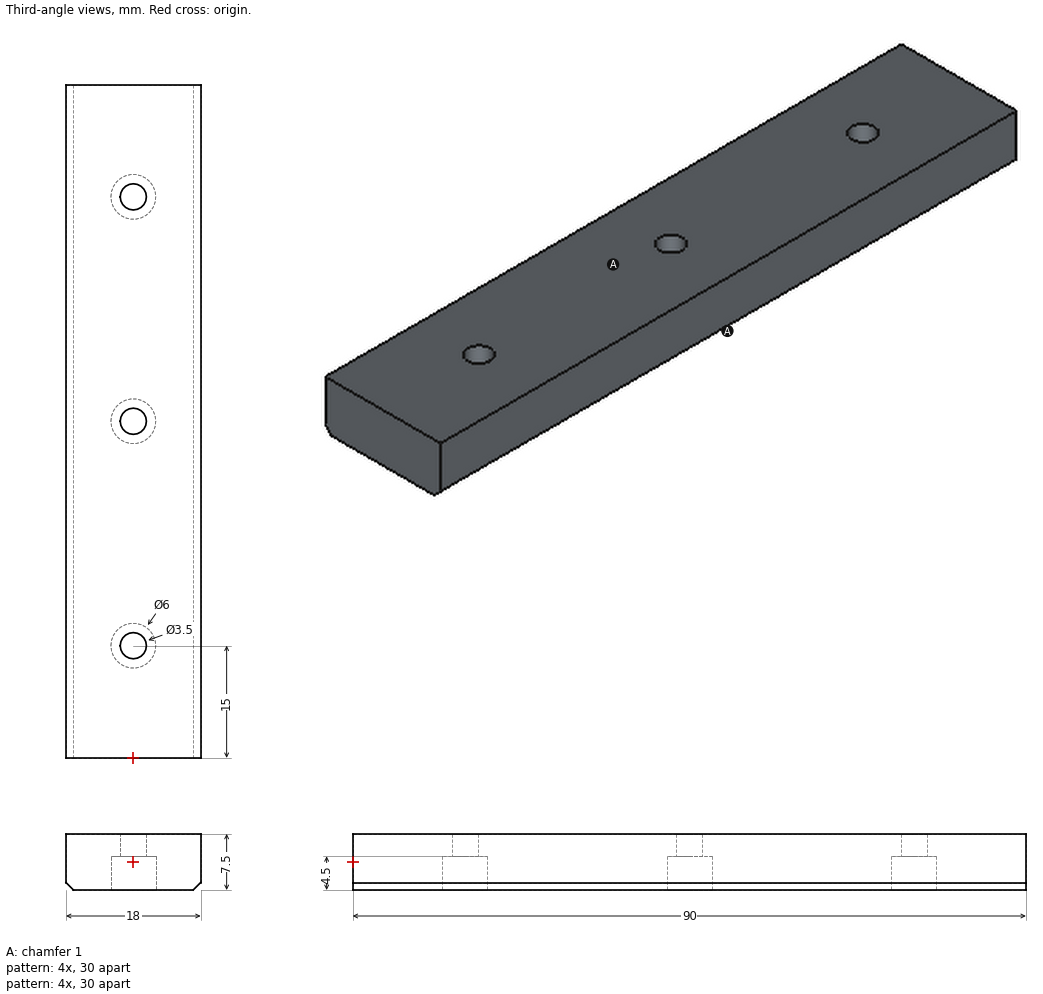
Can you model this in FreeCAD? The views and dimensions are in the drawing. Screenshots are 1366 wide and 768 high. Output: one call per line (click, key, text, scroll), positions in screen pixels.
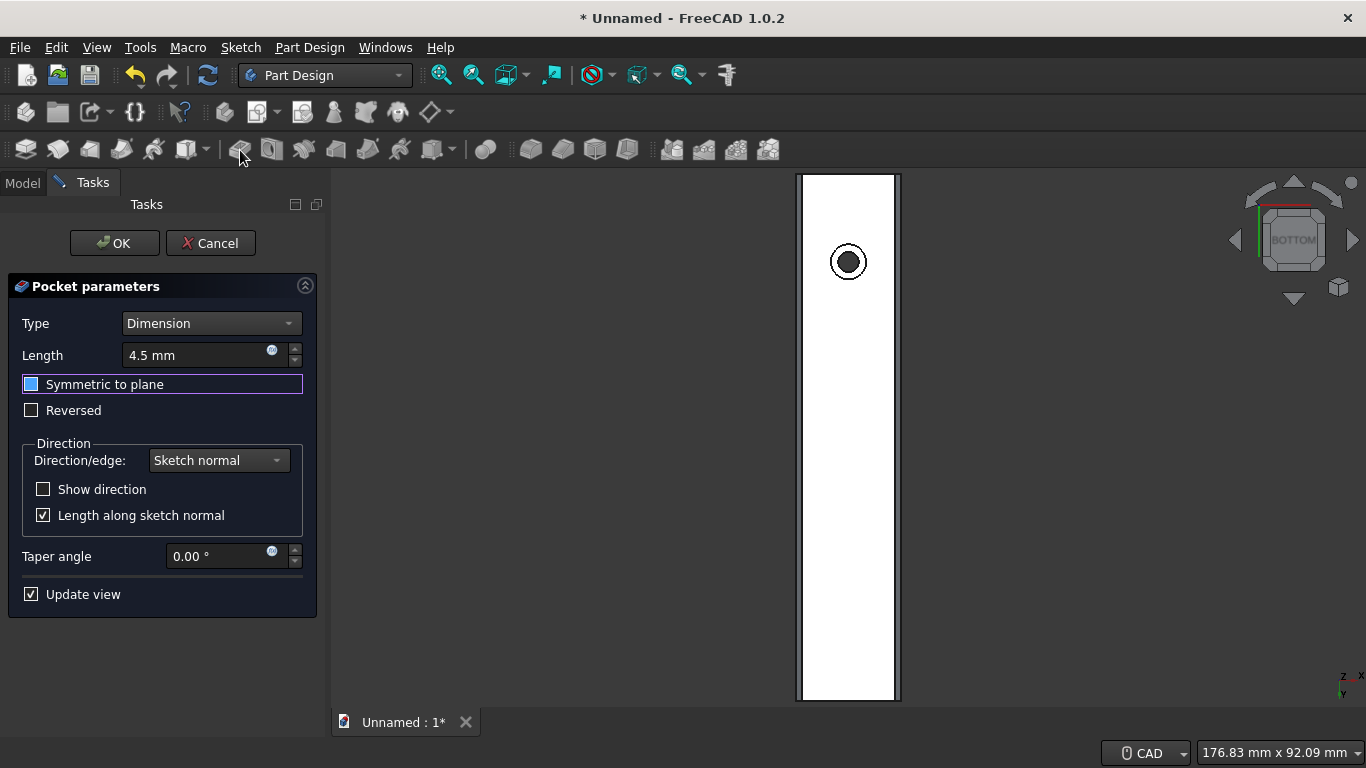
click(115, 243)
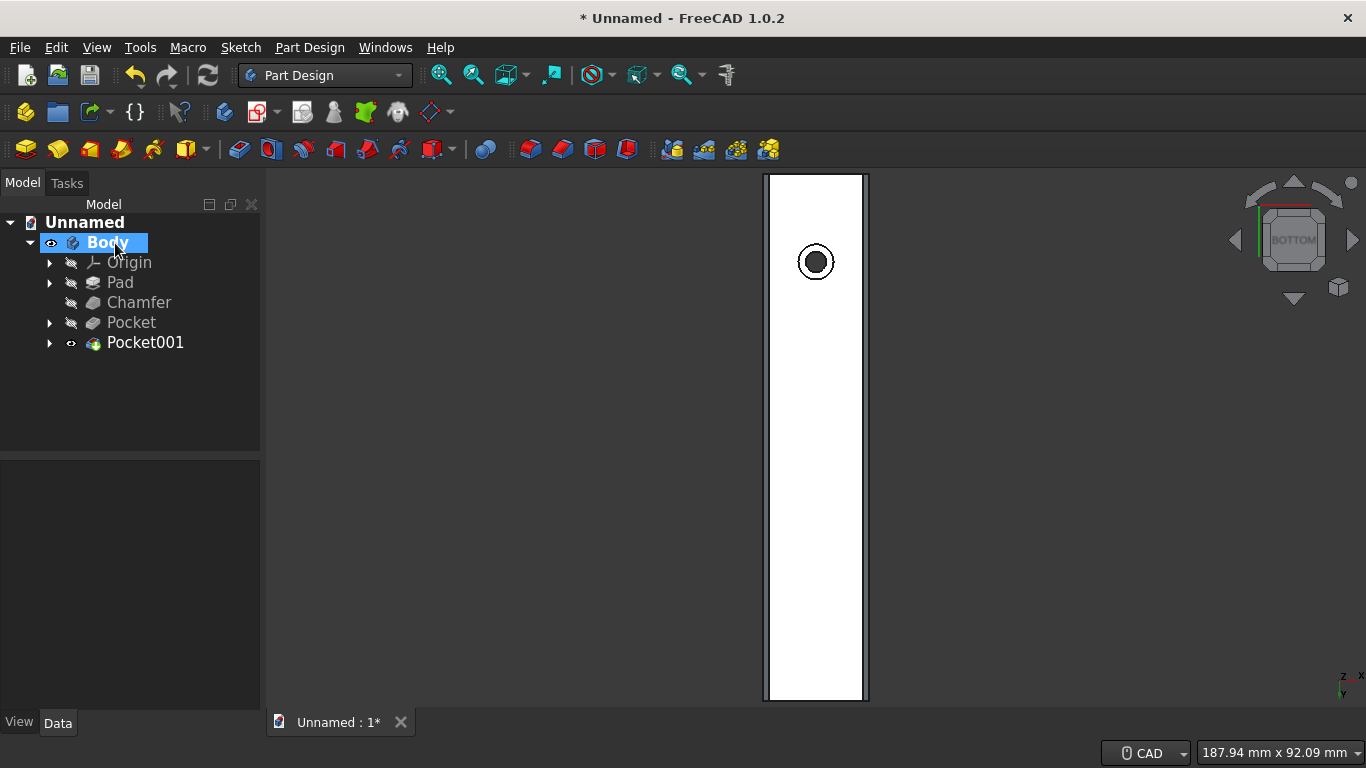
click(116, 343)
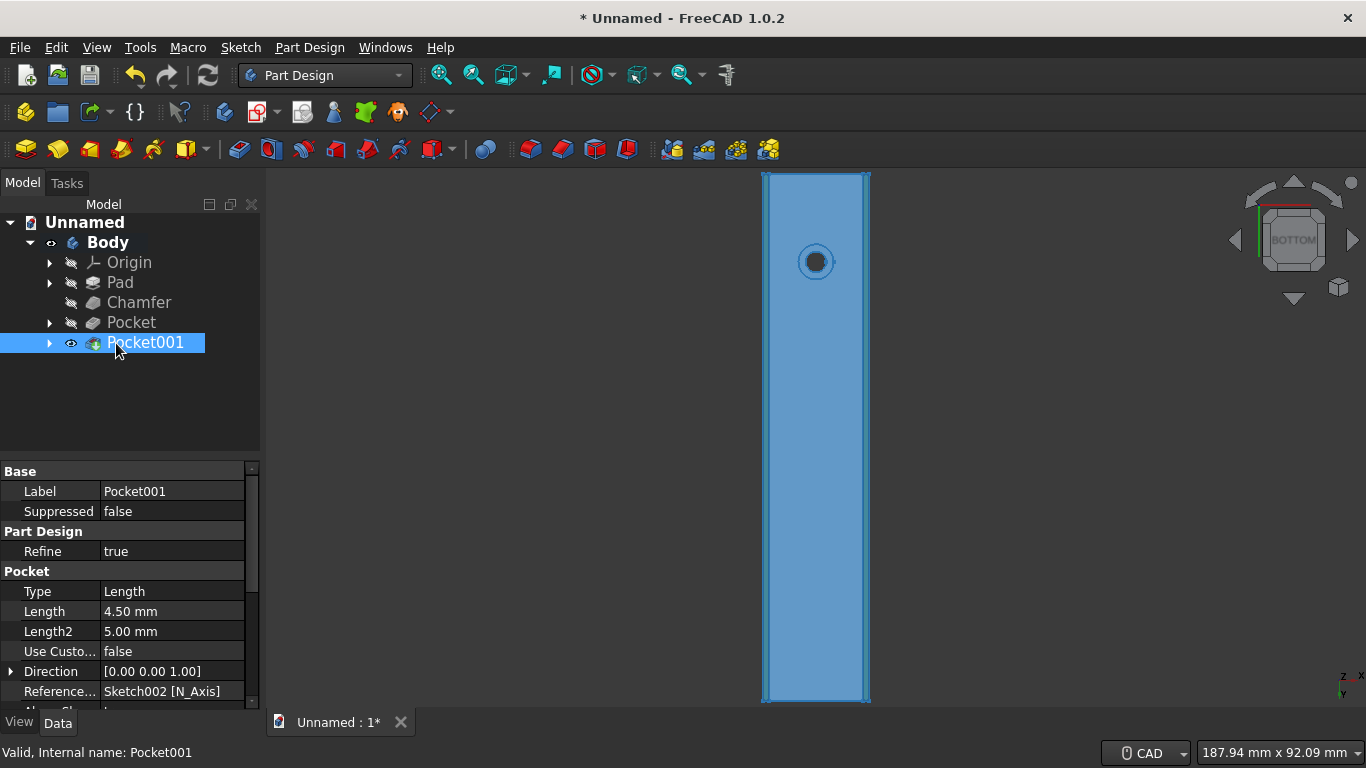
click(704, 150)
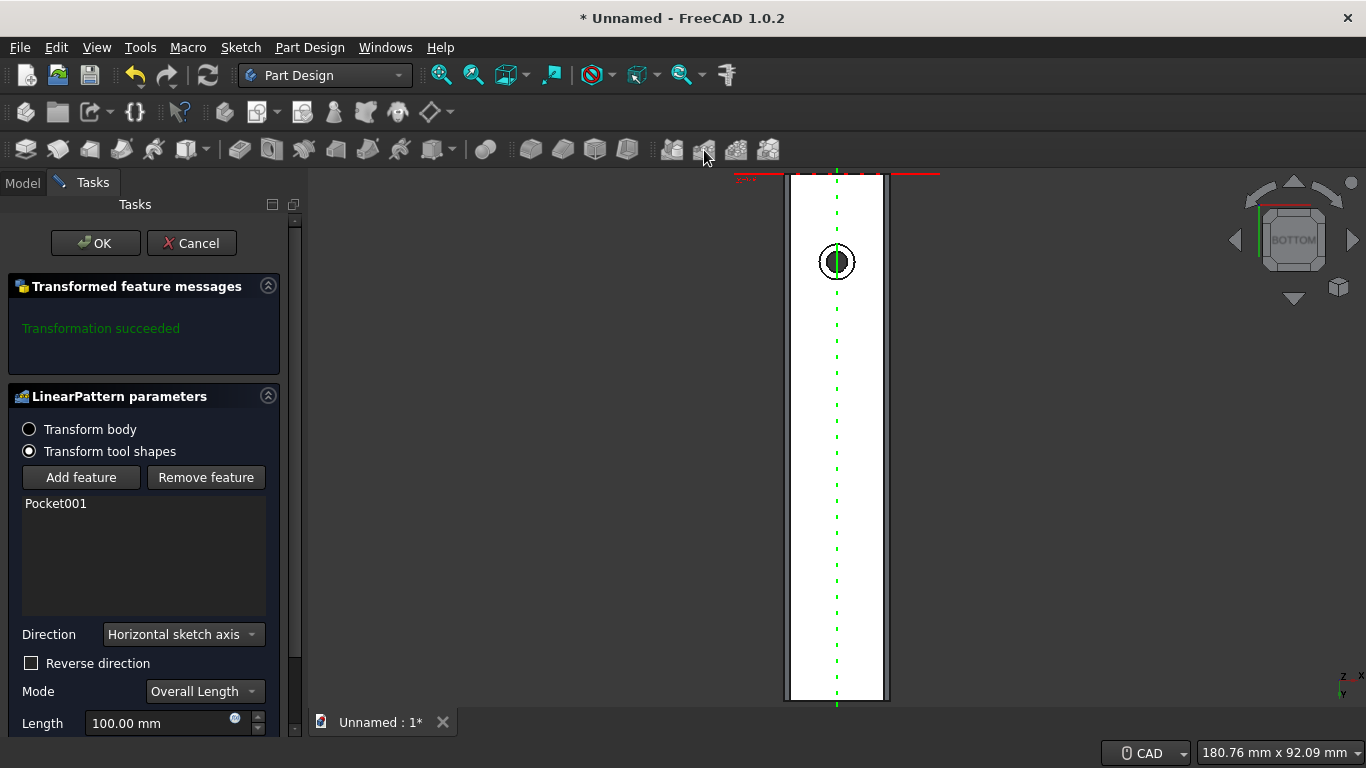
click(184, 634)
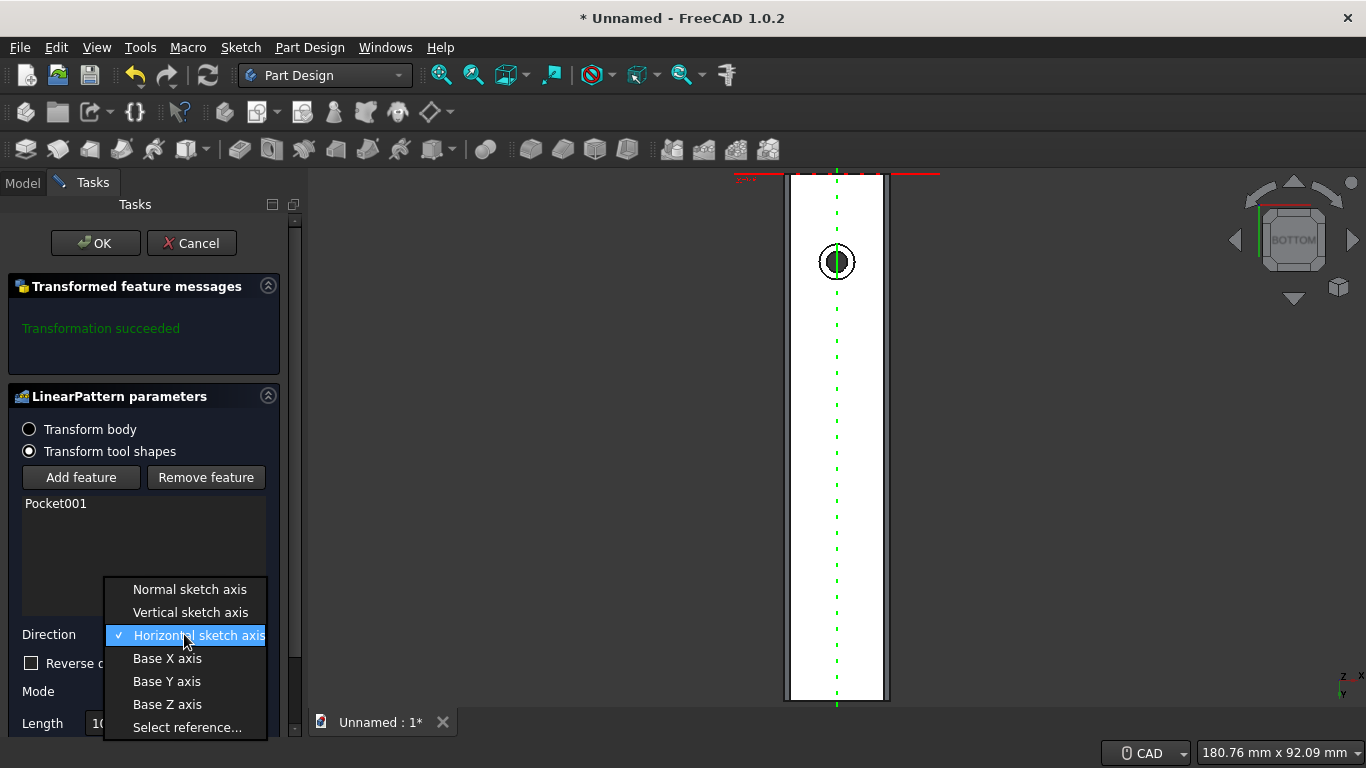
click(184, 682)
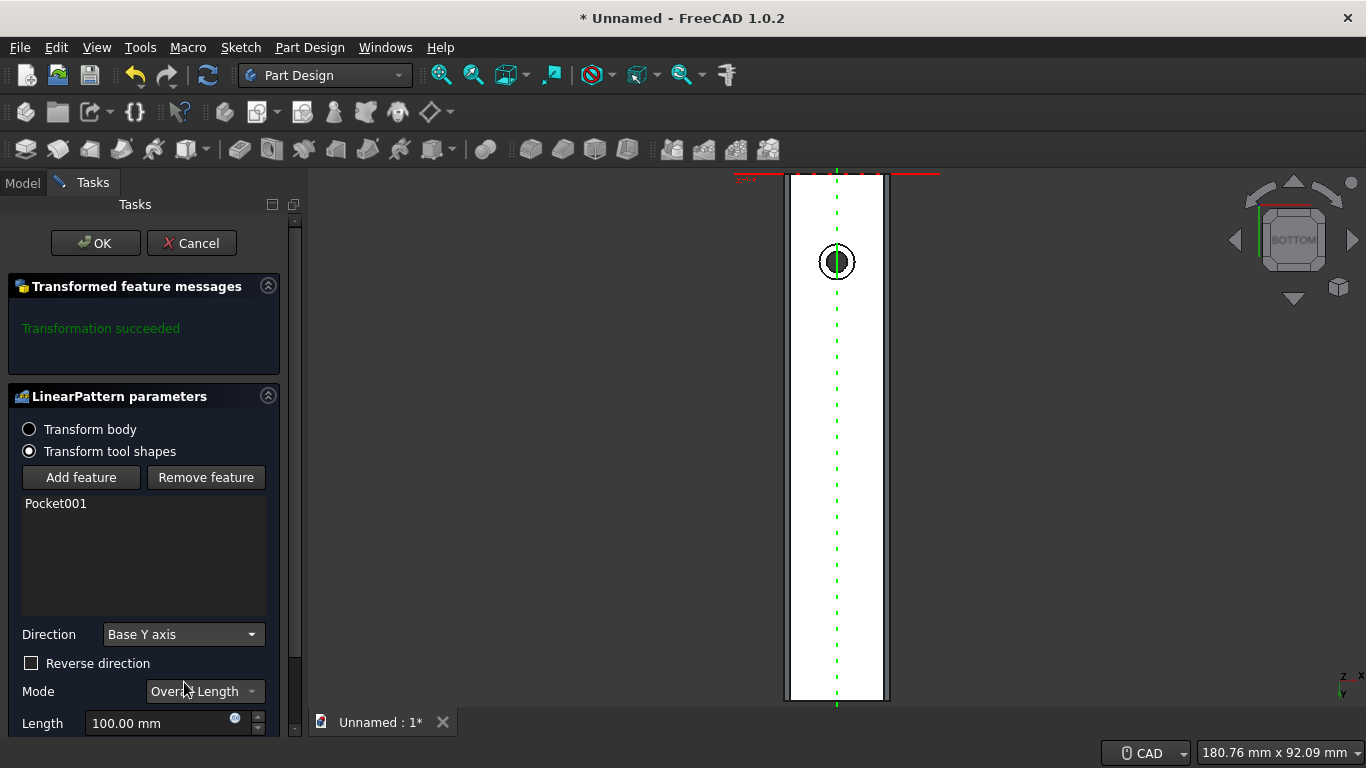
click(206, 692)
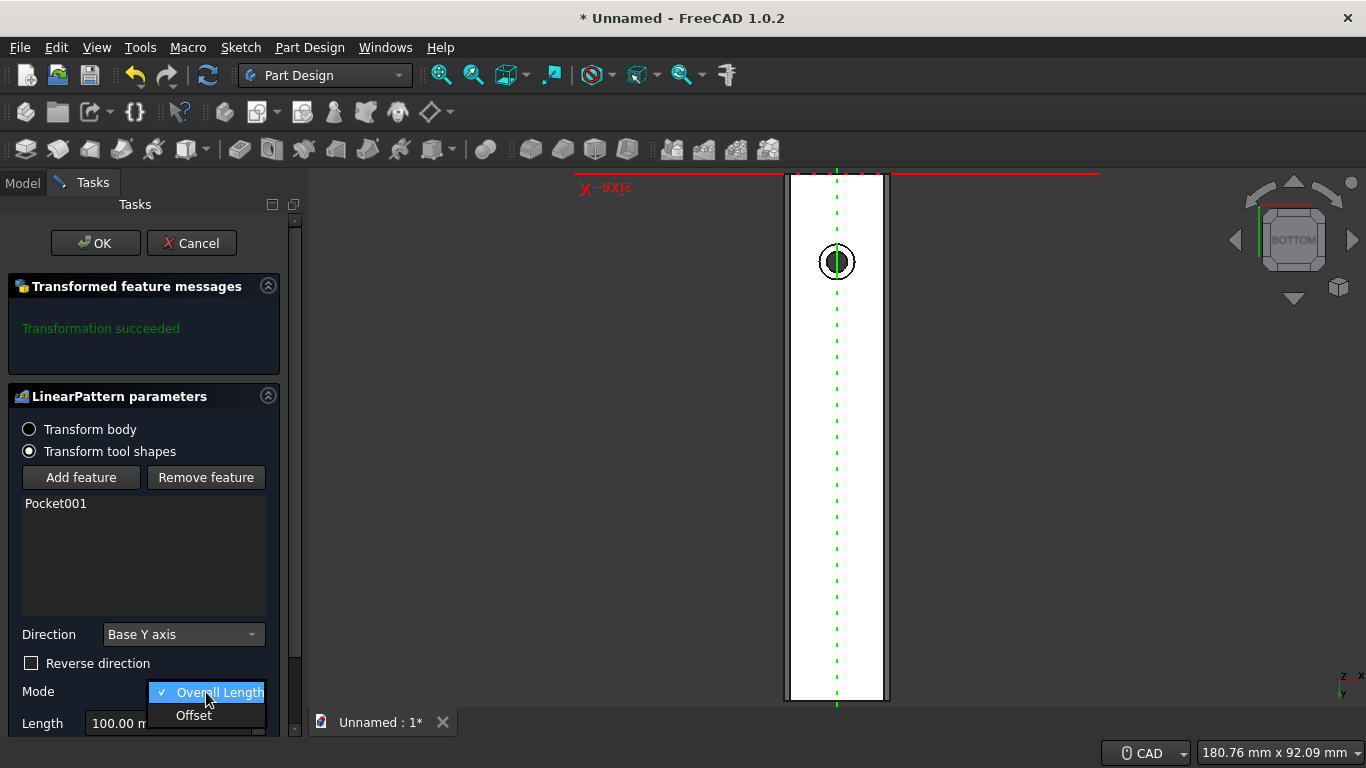
click(206, 716)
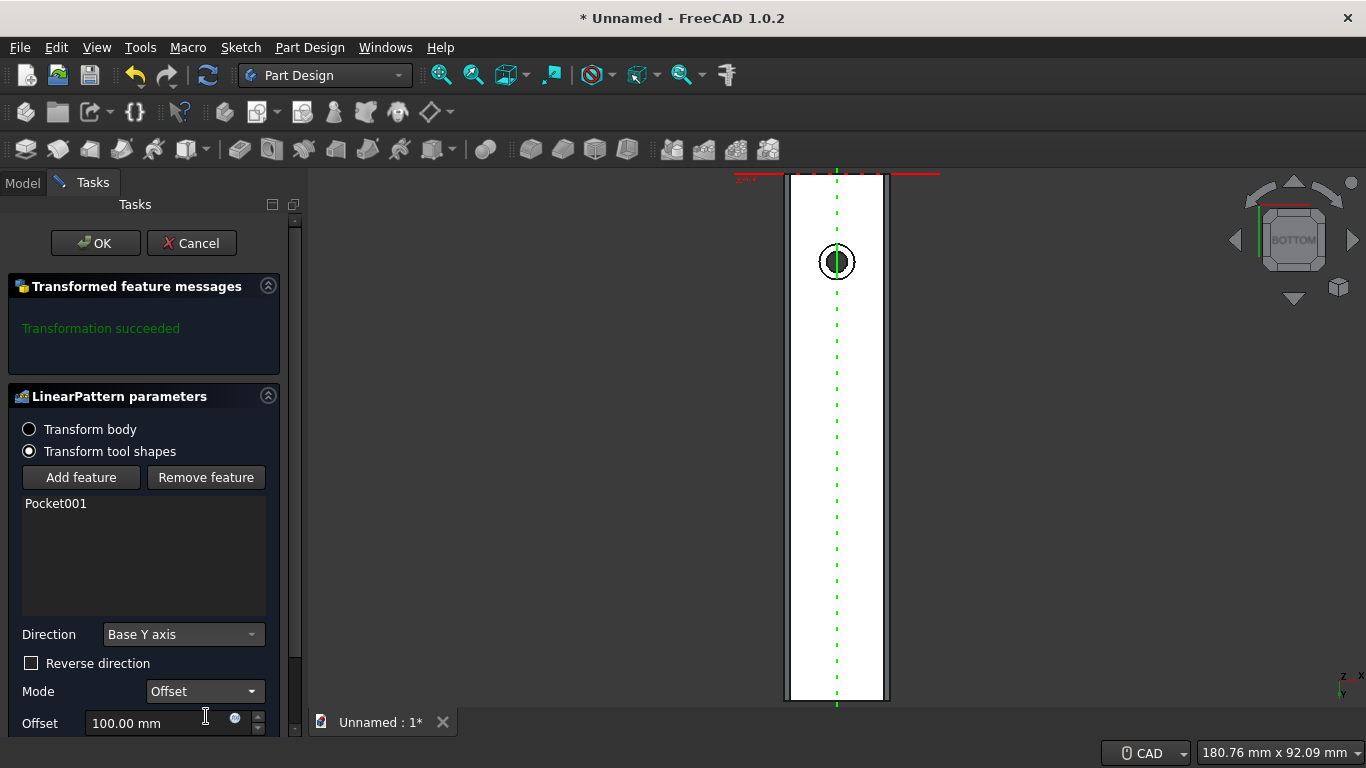
triple_click(168, 723)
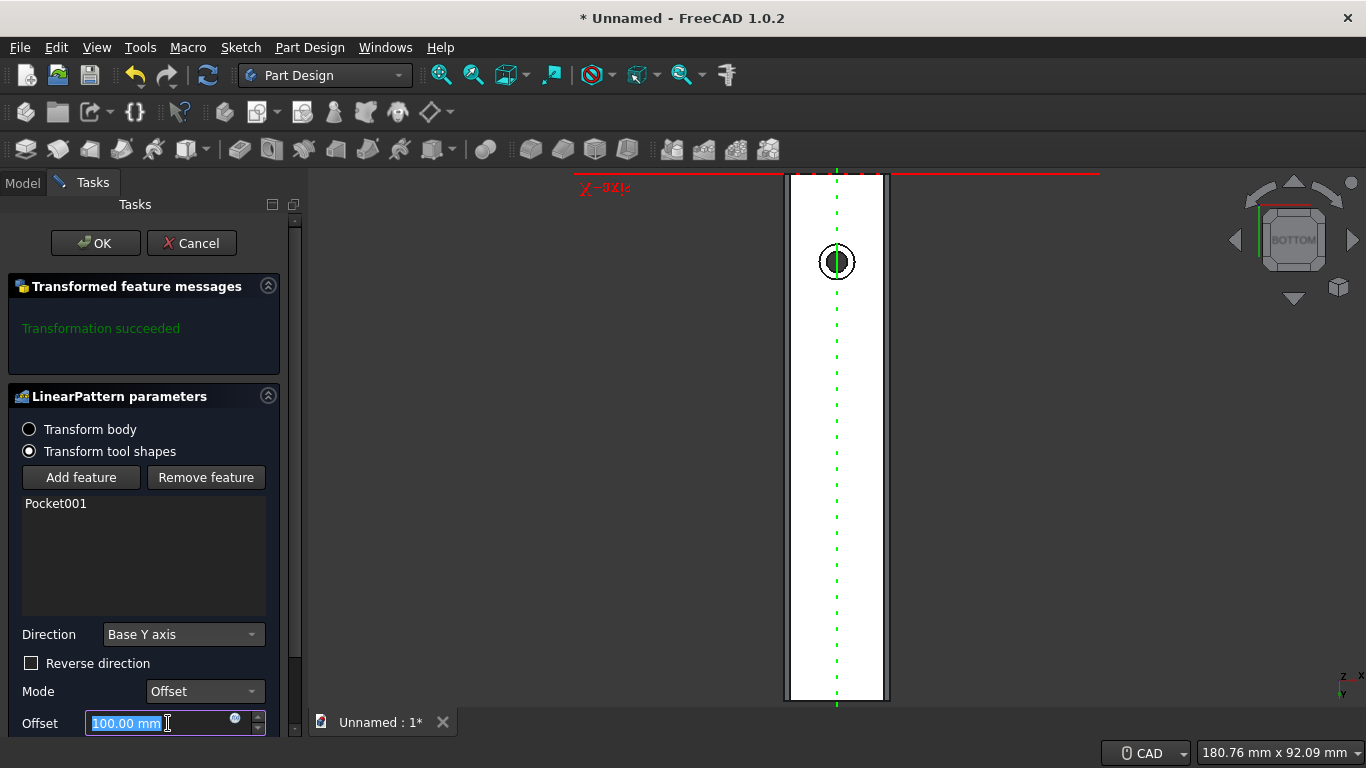
text(30)
key(Tab)